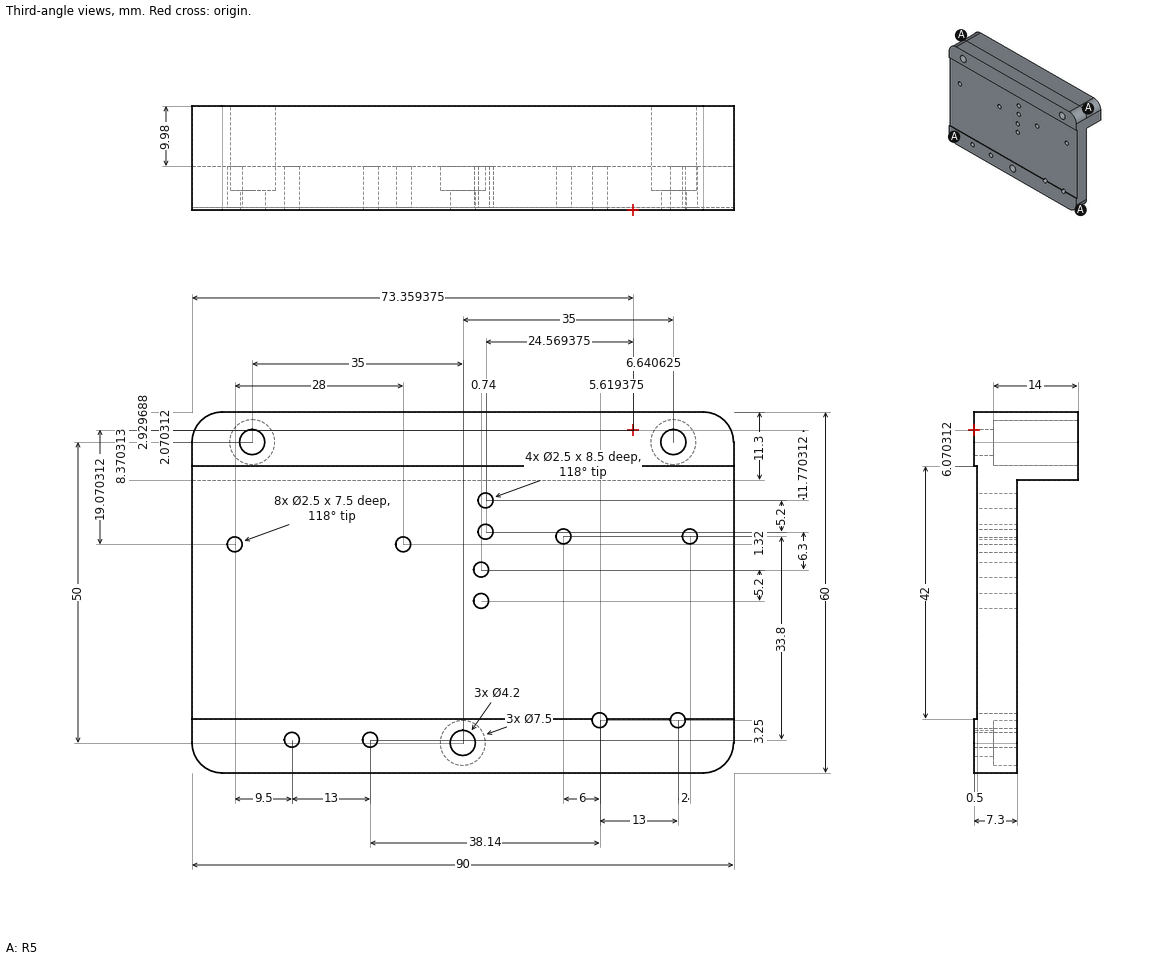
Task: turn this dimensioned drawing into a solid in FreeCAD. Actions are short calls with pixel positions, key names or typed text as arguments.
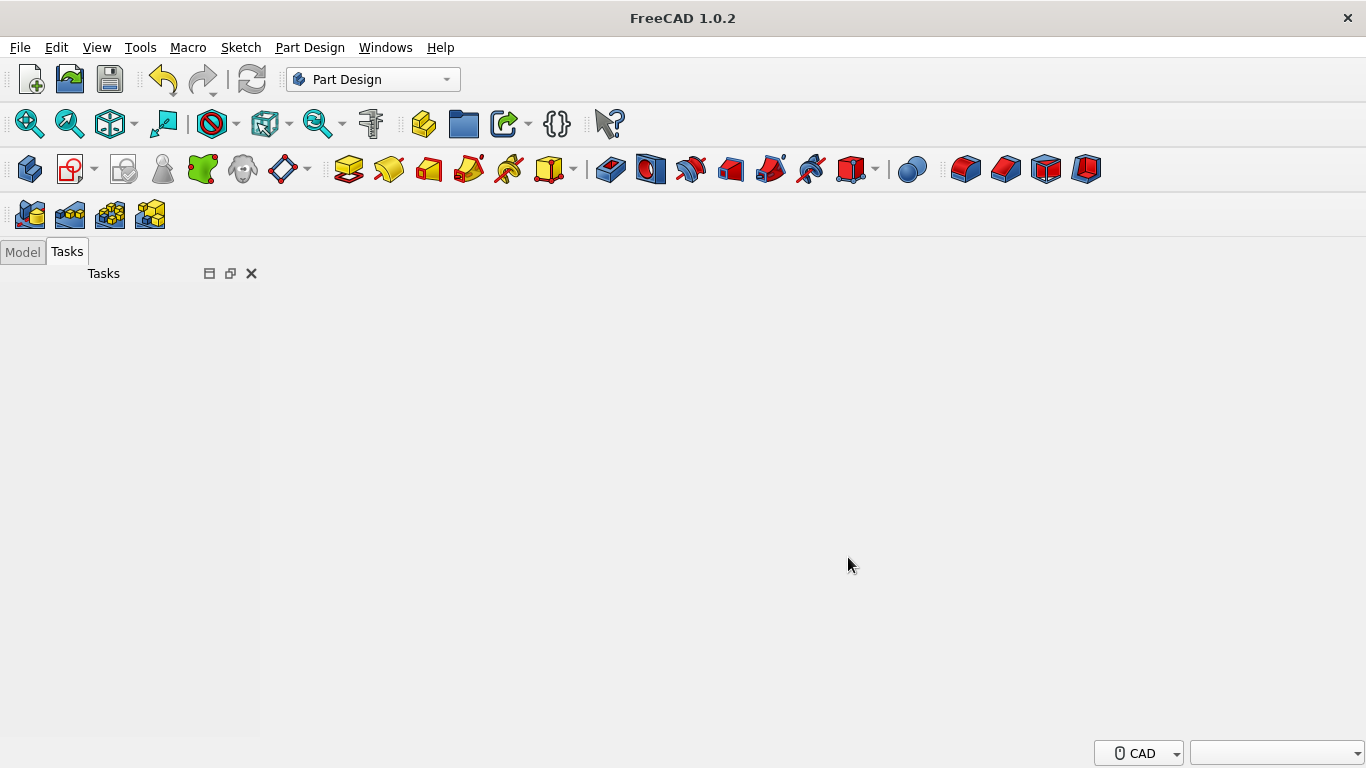
click(30, 80)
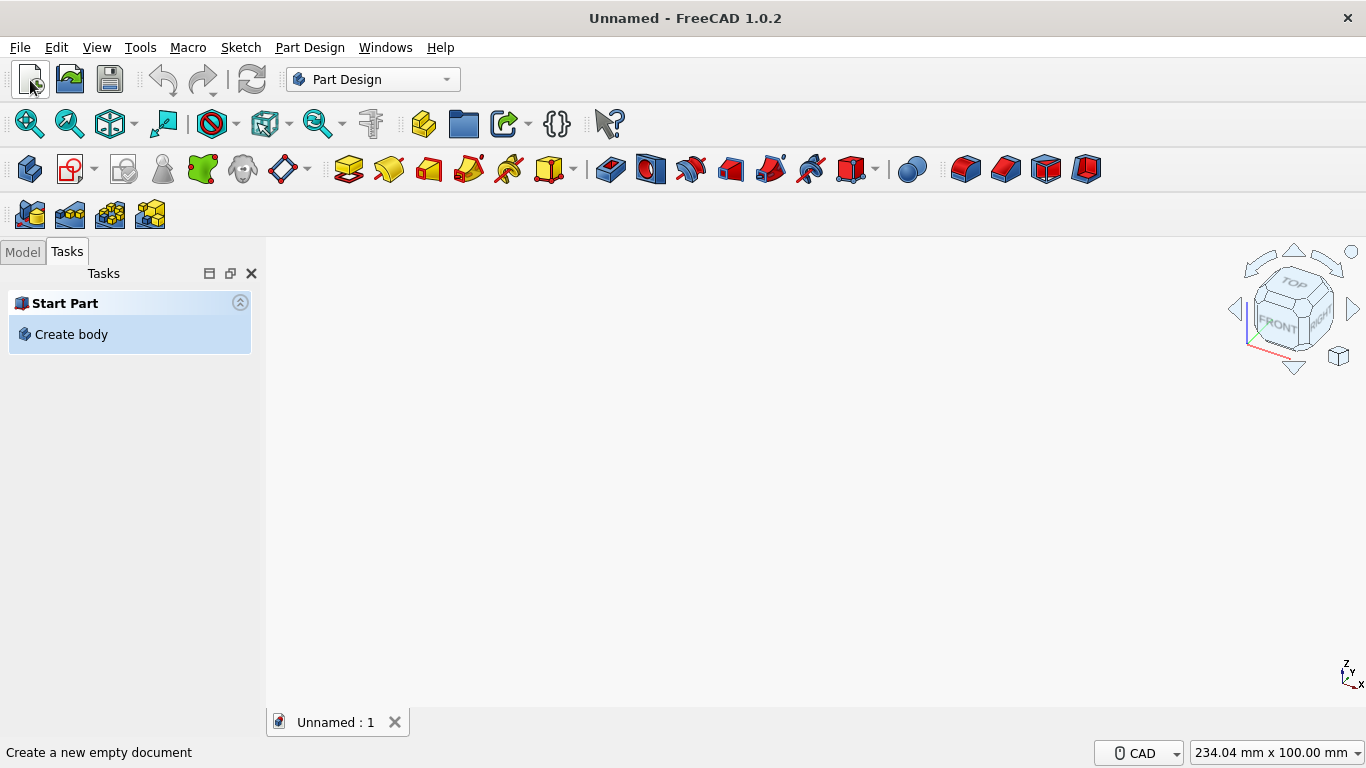
click(70, 170)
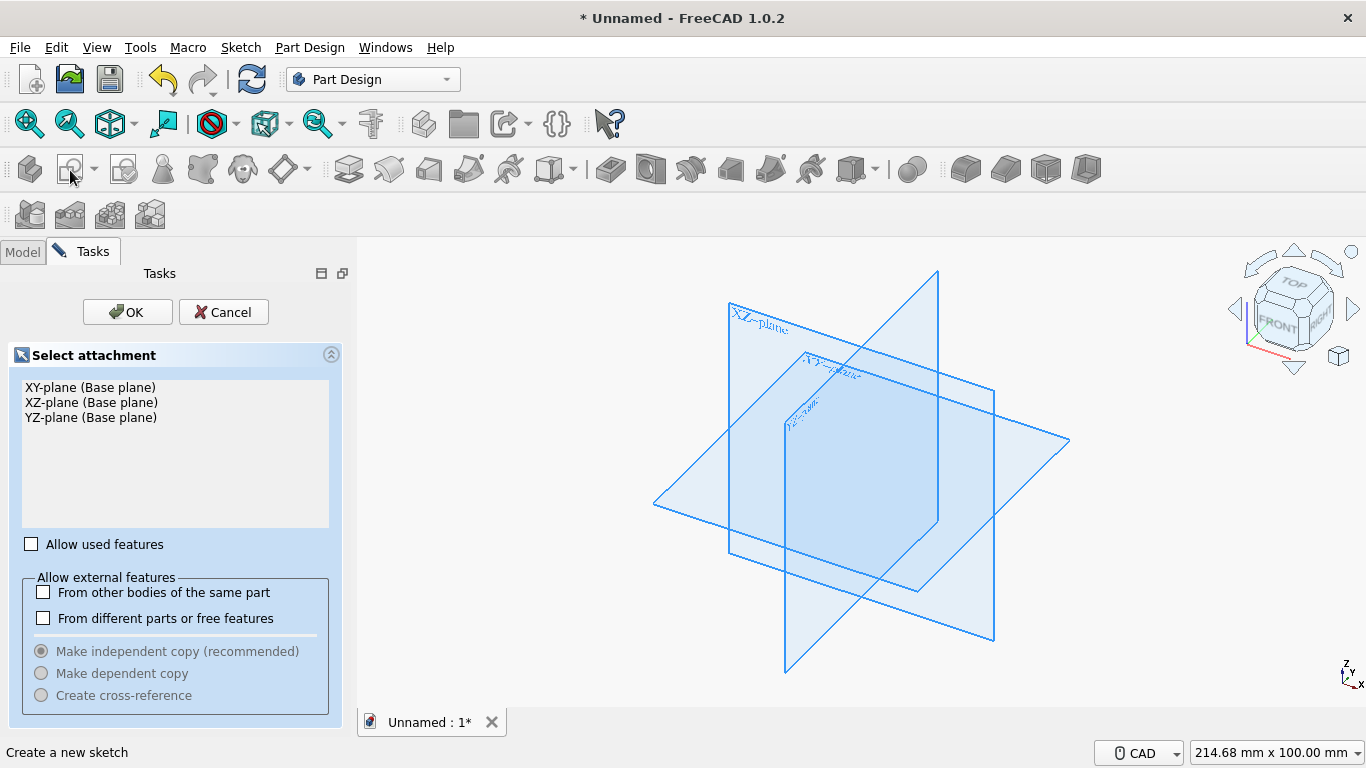
click(82, 402)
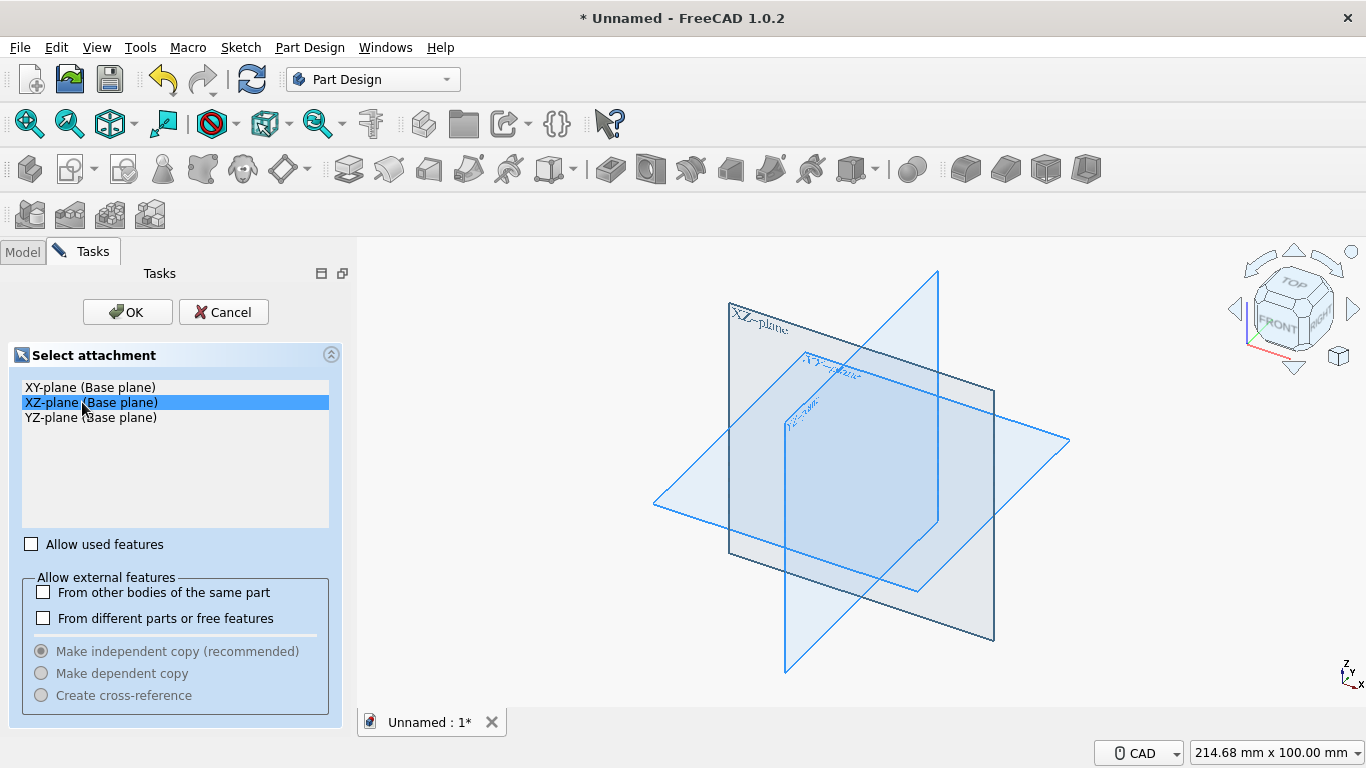
click(128, 312)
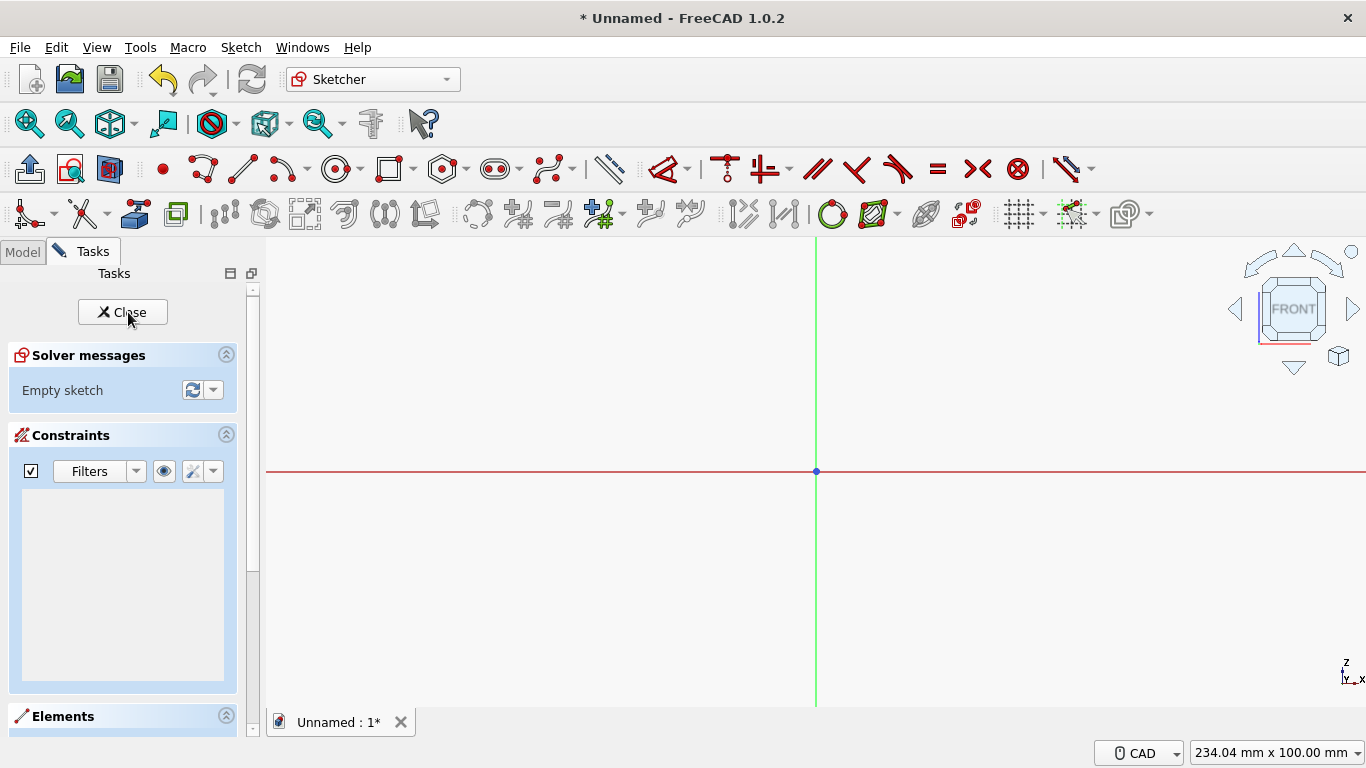
scroll(879, 265, down, 2)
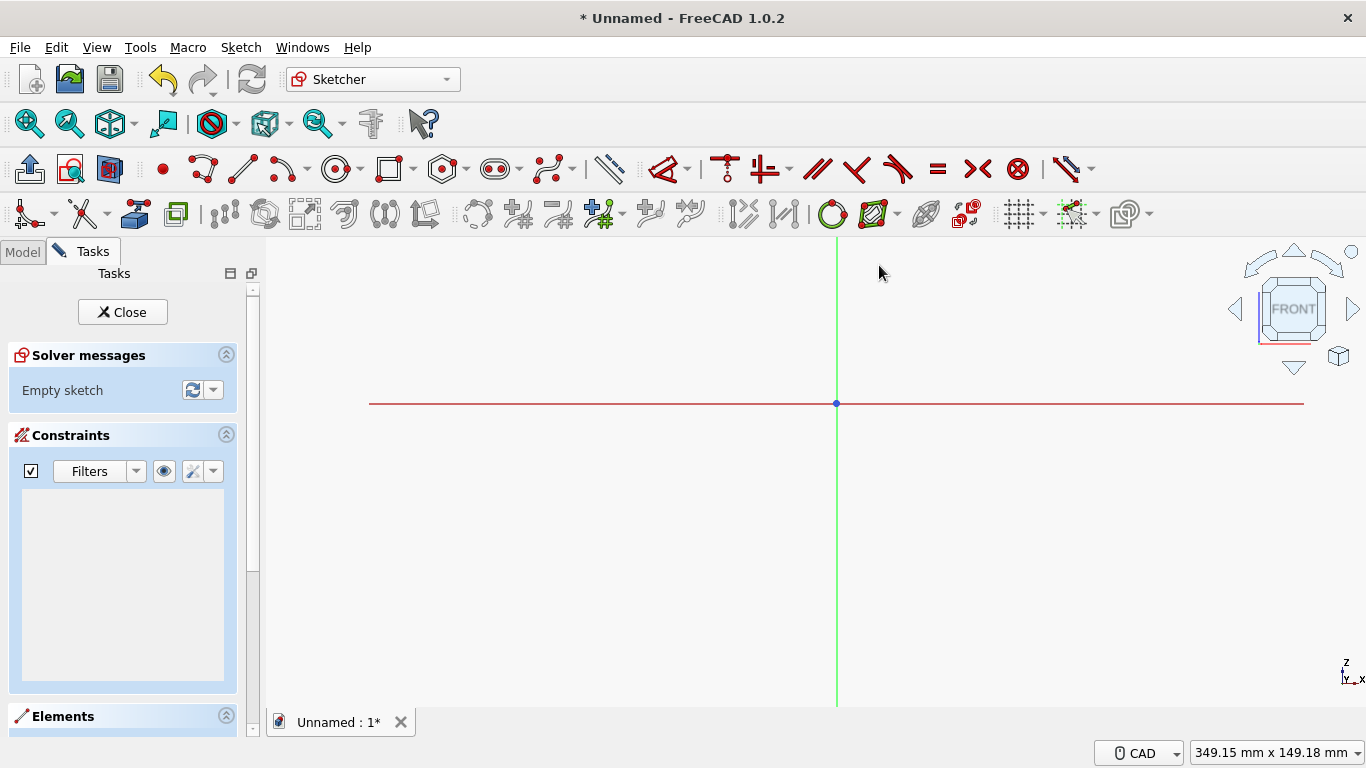
scroll(748, 524, up, 2)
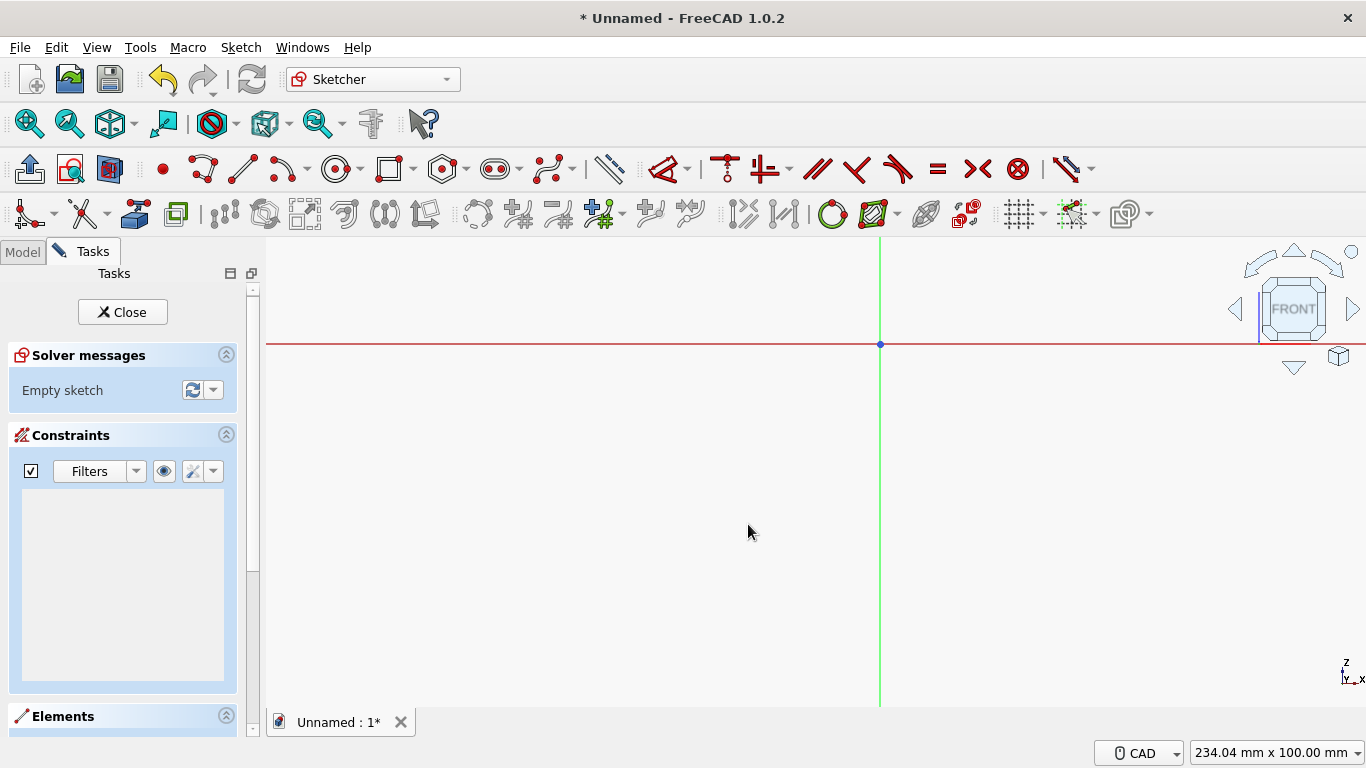
click(390, 170)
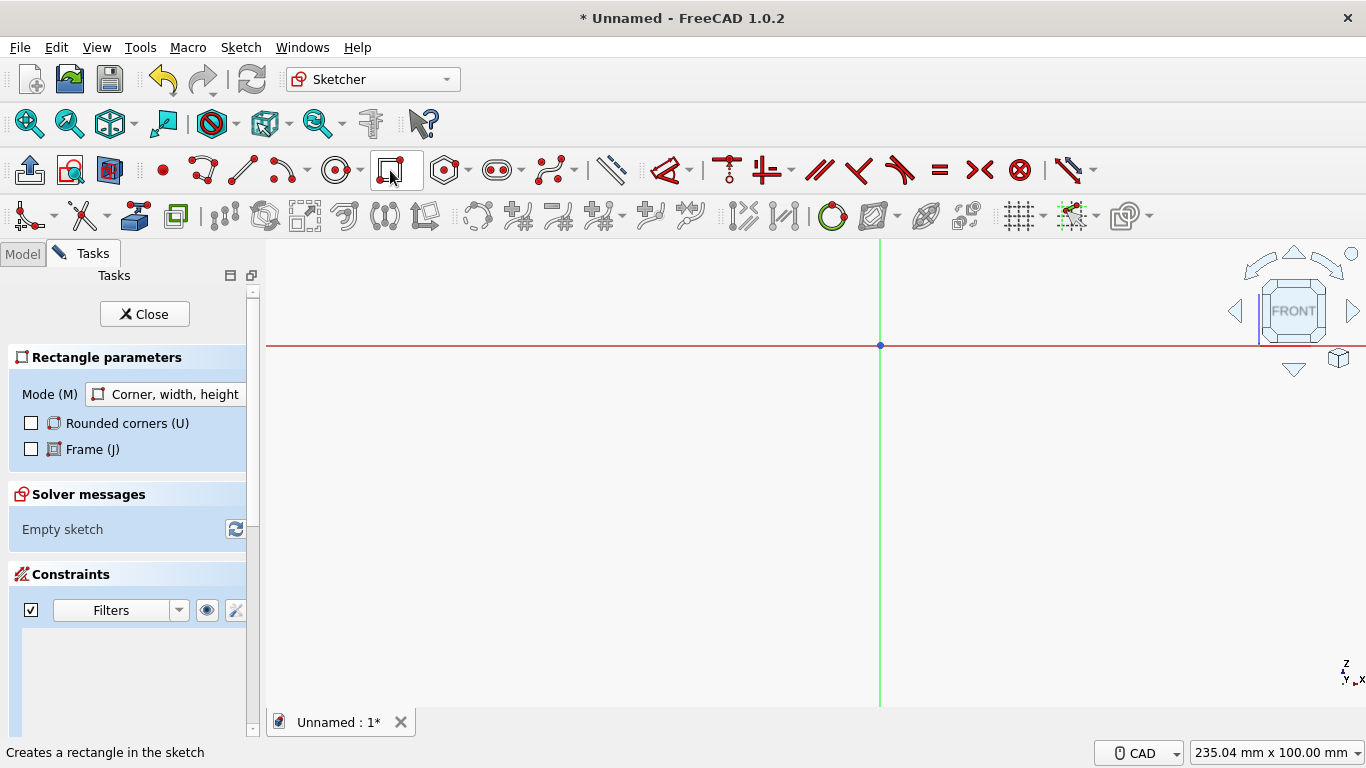
click(537, 332)
move(958, 613)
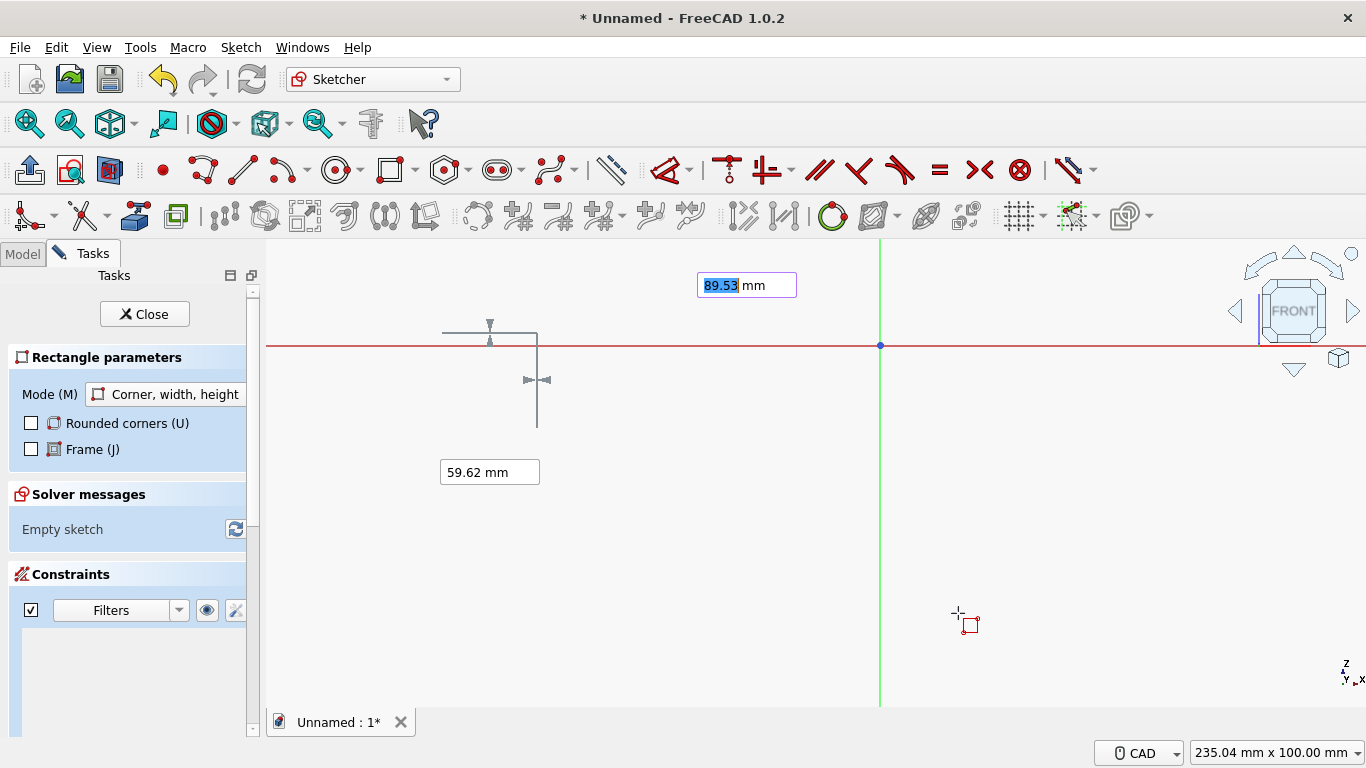
text(90)
key(Tab)
text(60)
key(Return)
key(Escape)